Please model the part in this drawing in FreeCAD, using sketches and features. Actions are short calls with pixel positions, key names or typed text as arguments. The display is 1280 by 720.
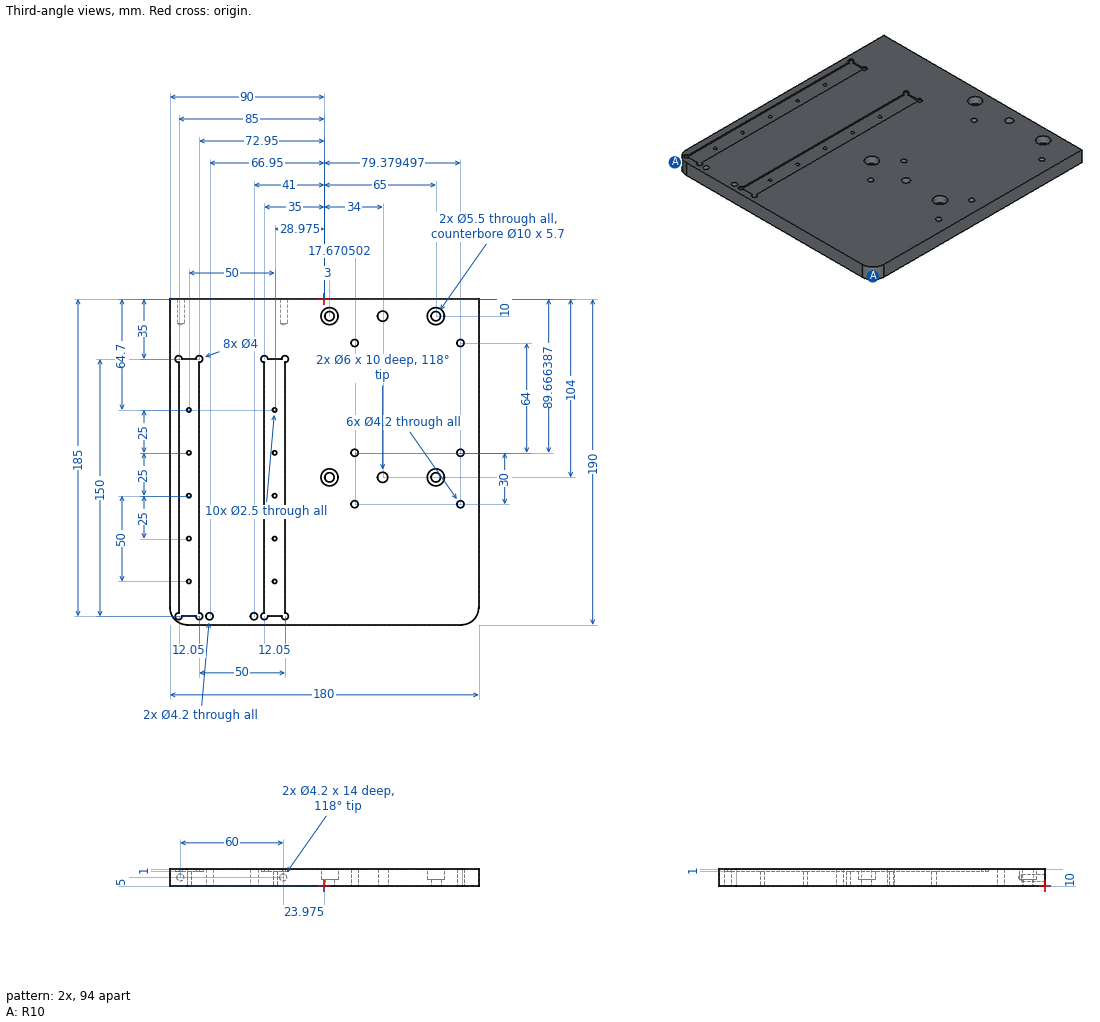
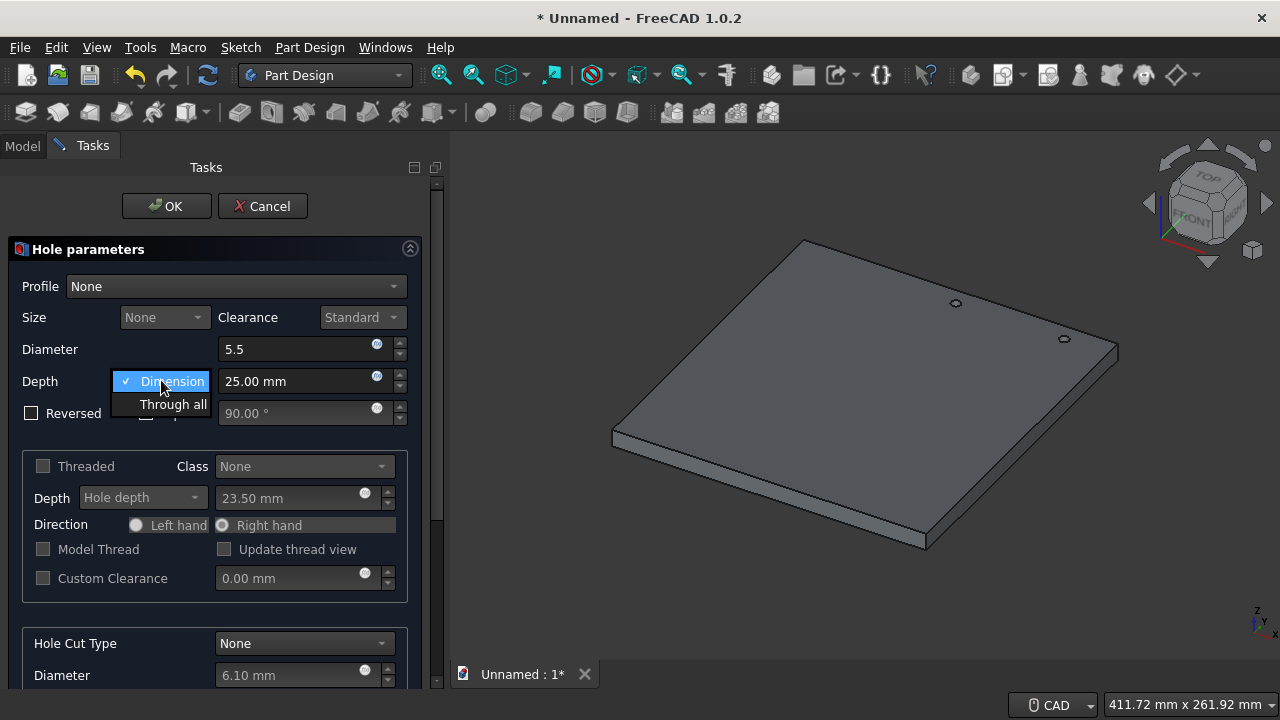
click(160, 404)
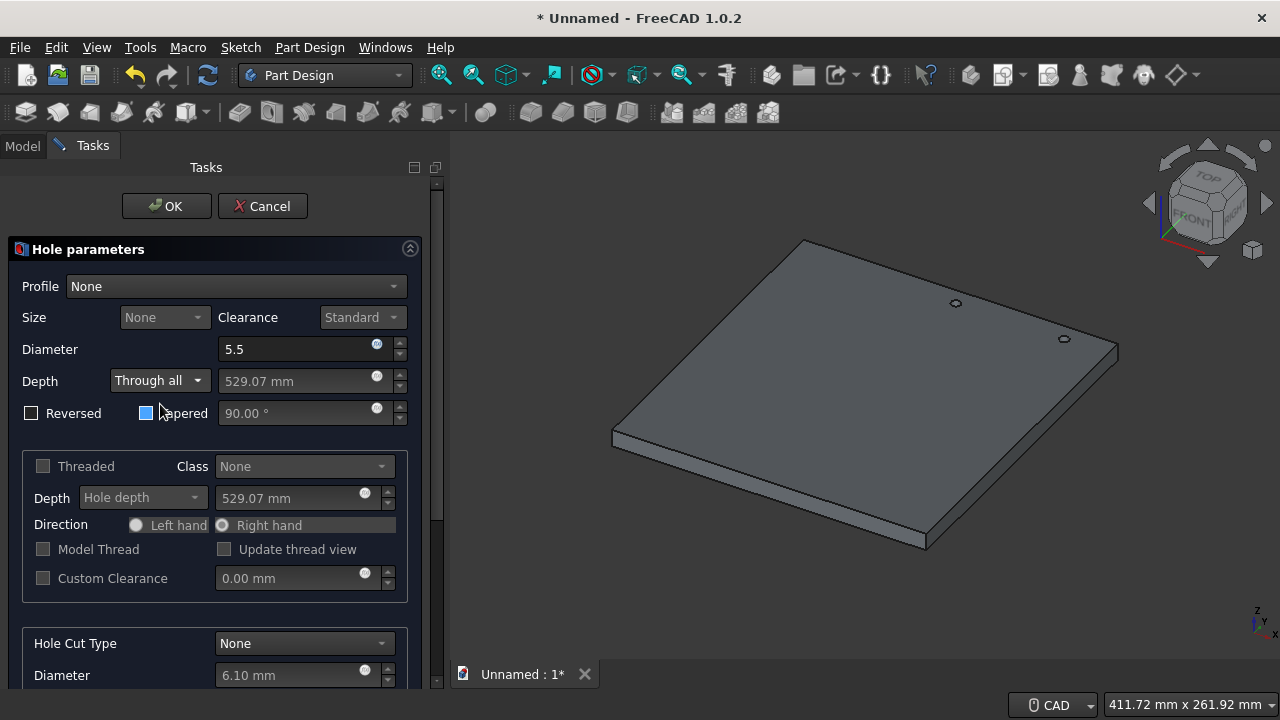
click(306, 644)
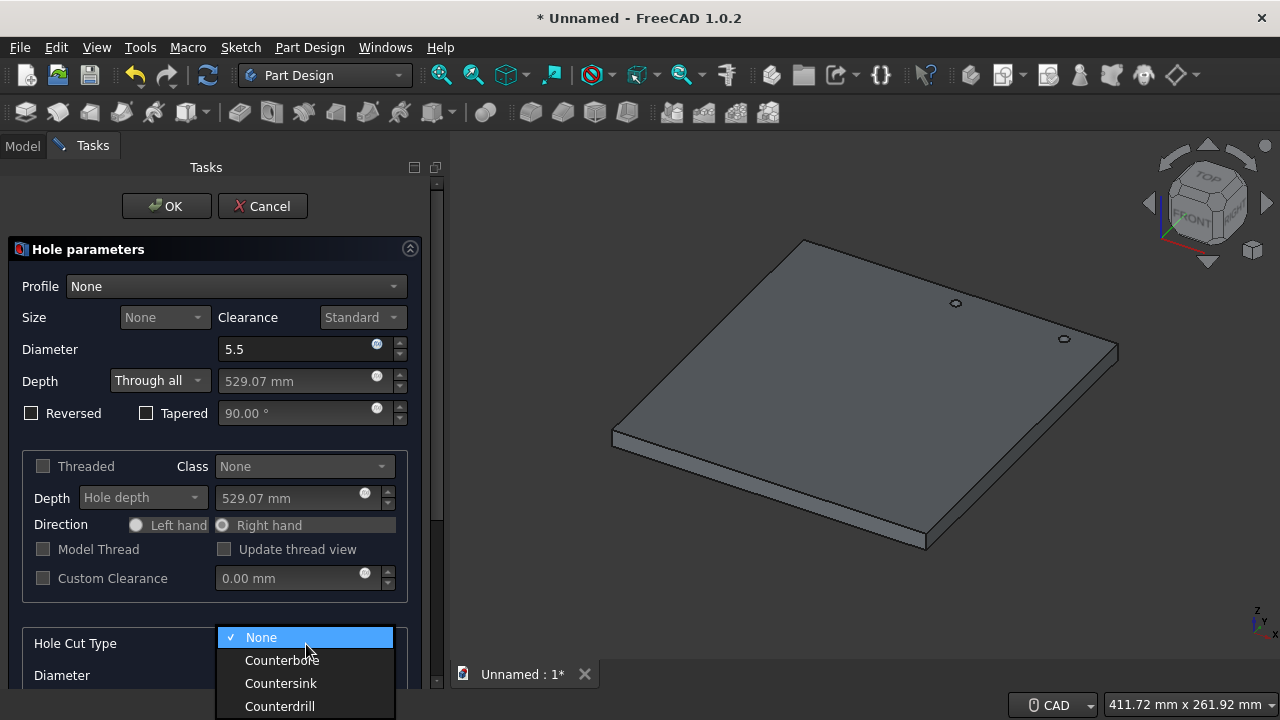
click(304, 660)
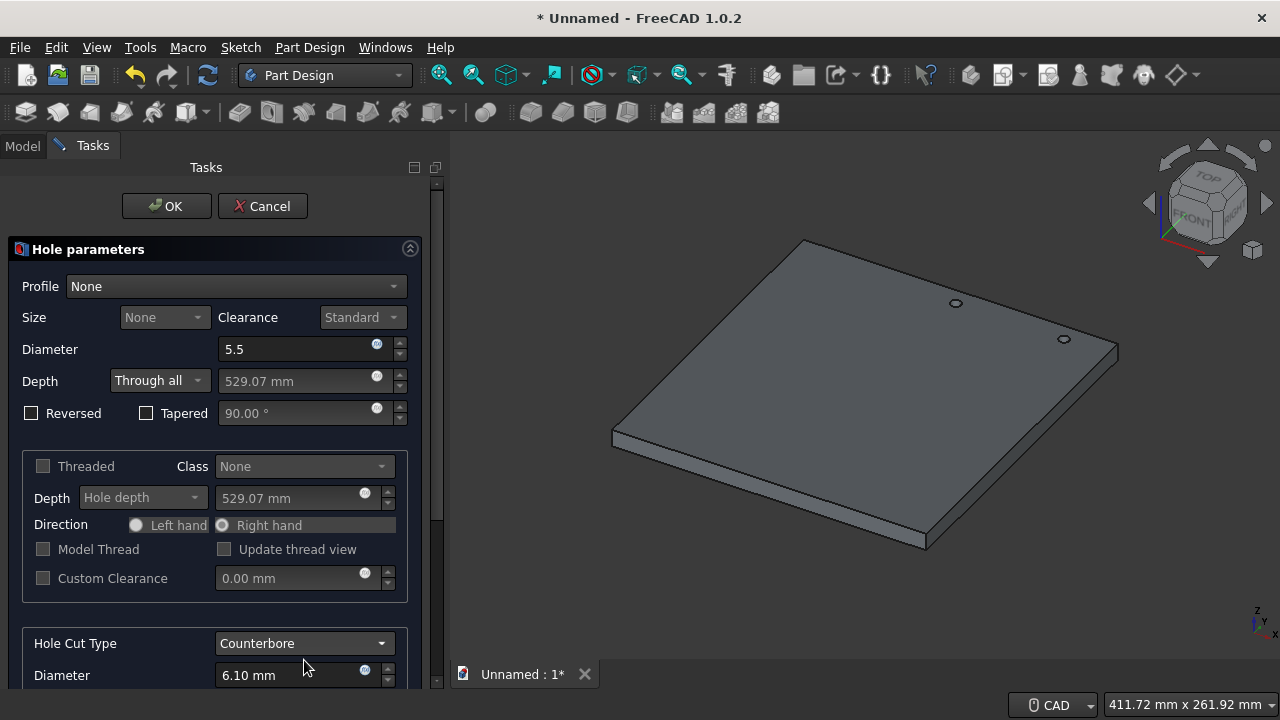
triple_click(298, 675)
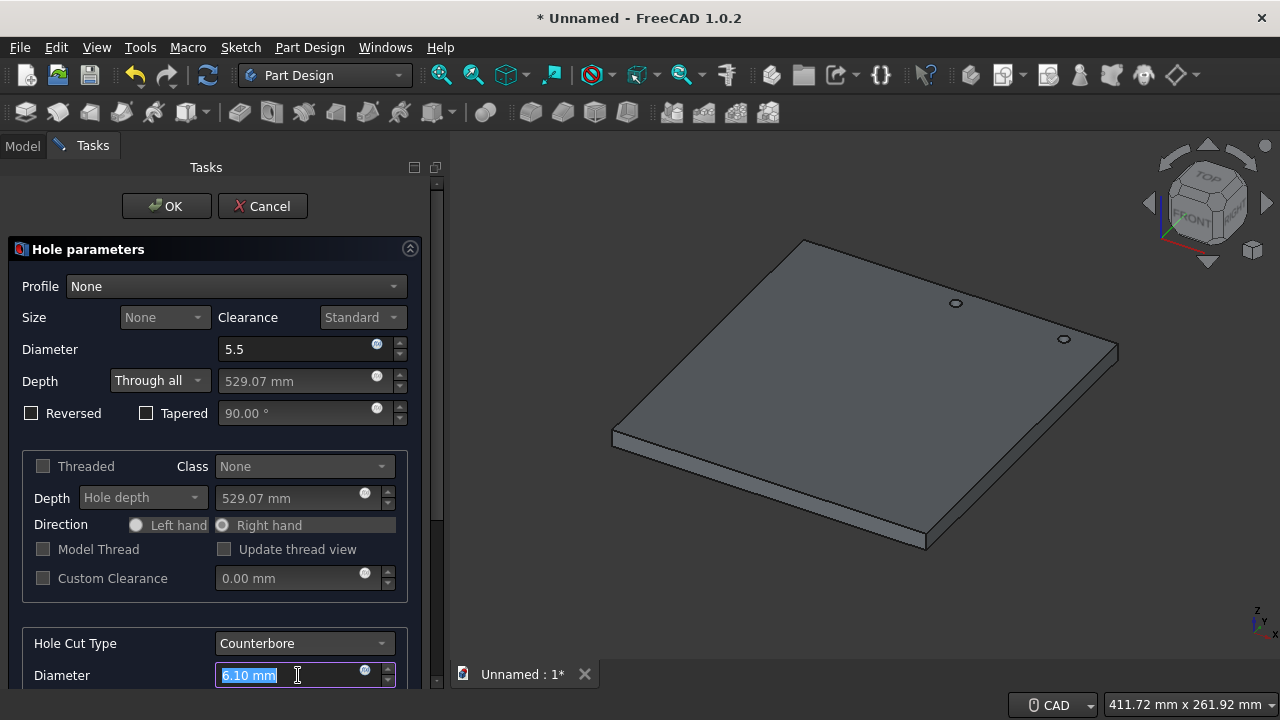
text(10)
key(Tab)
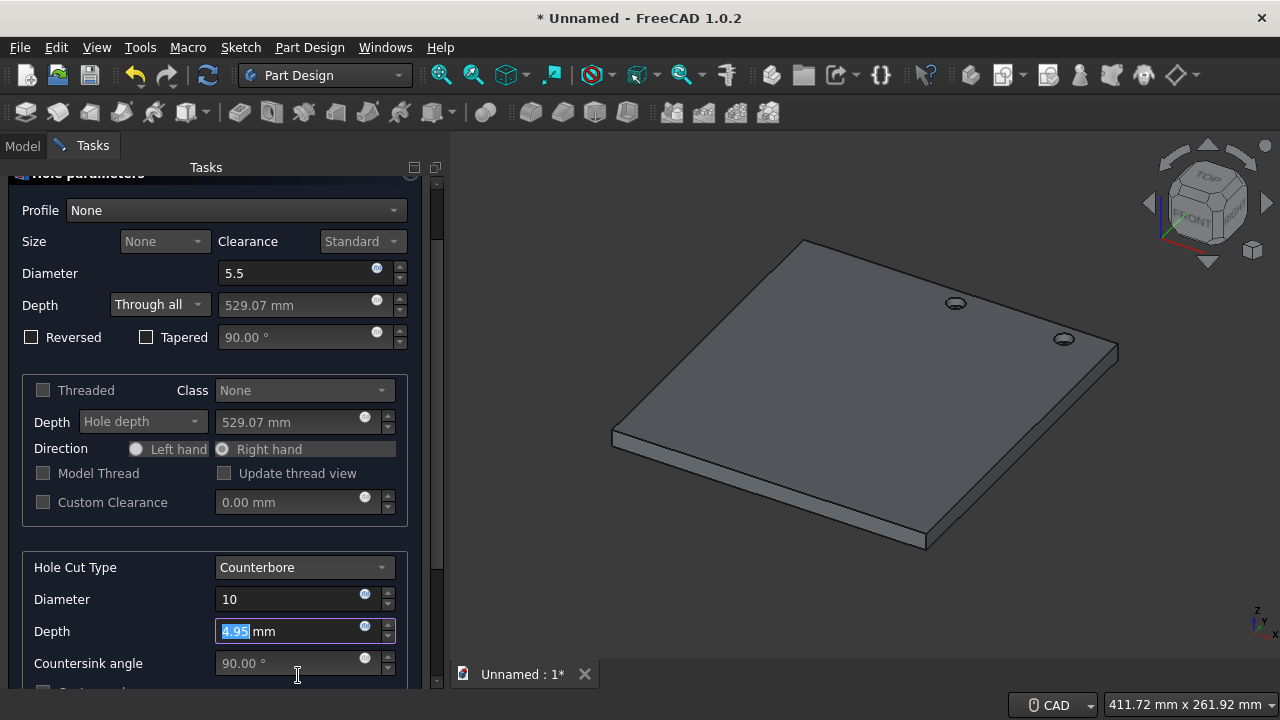
text(5.7)
key(Tab)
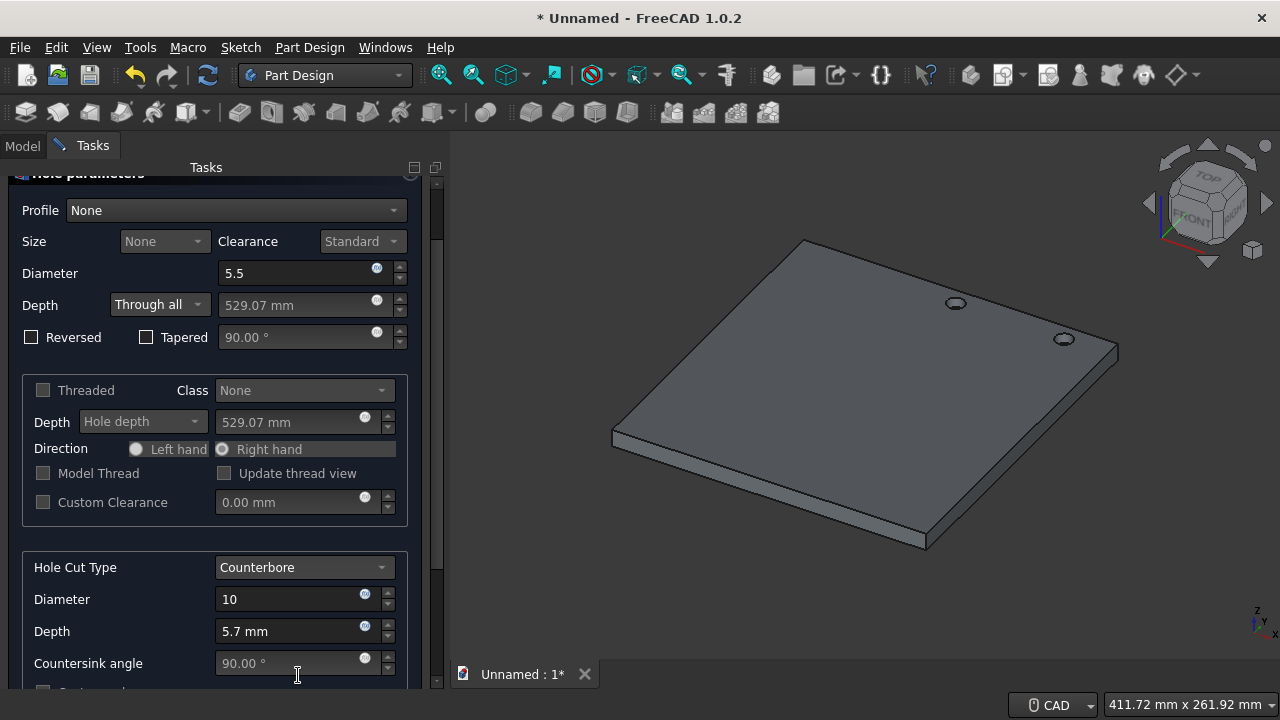
scroll(437, 432, up, 3)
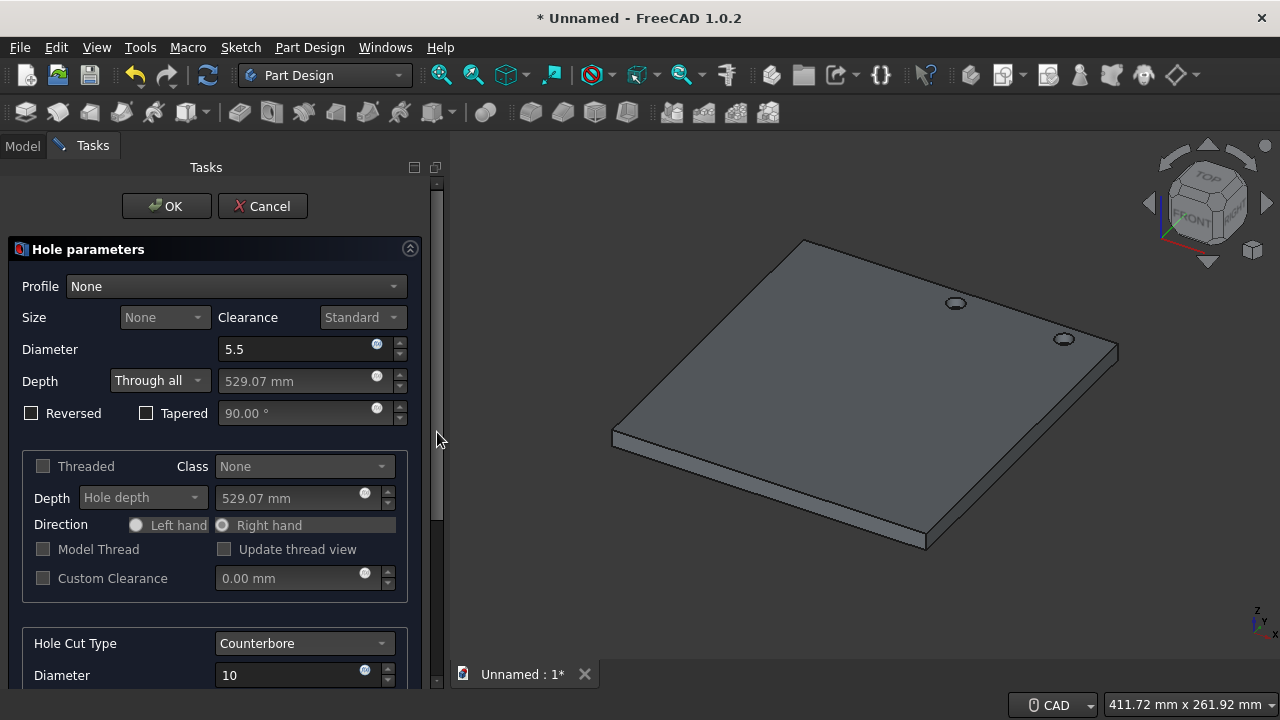
click(167, 206)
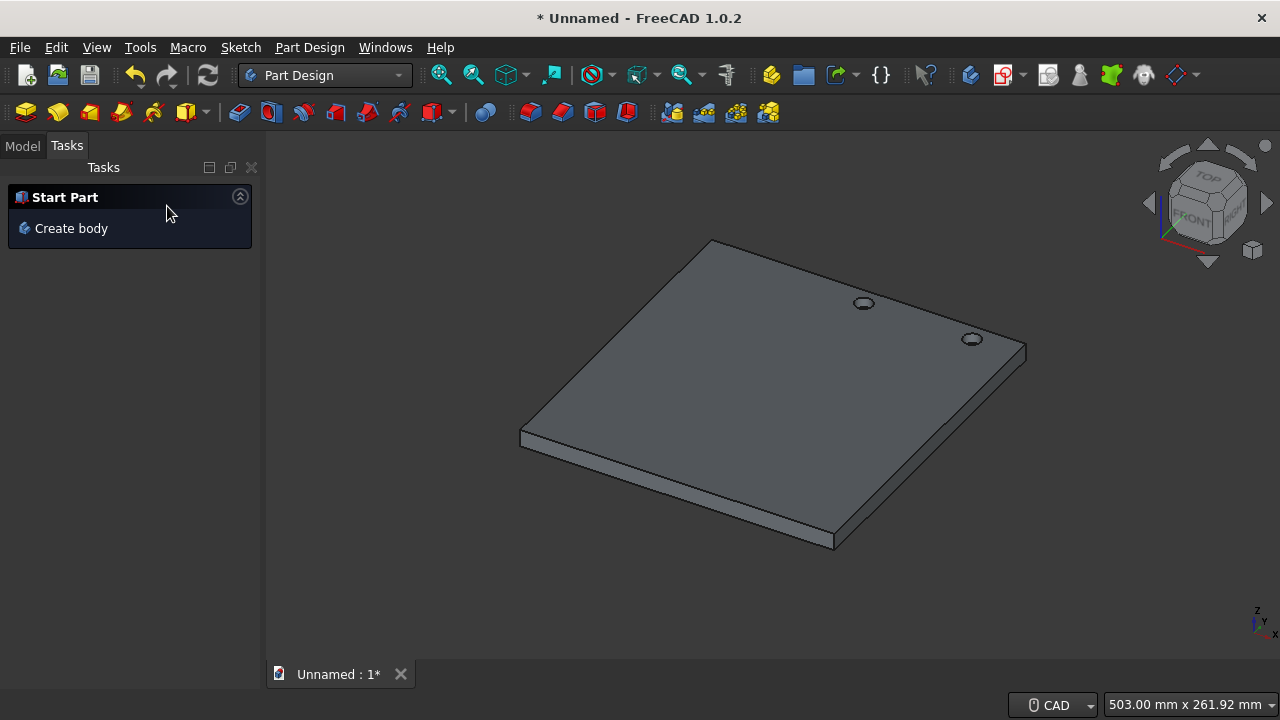
click(23, 145)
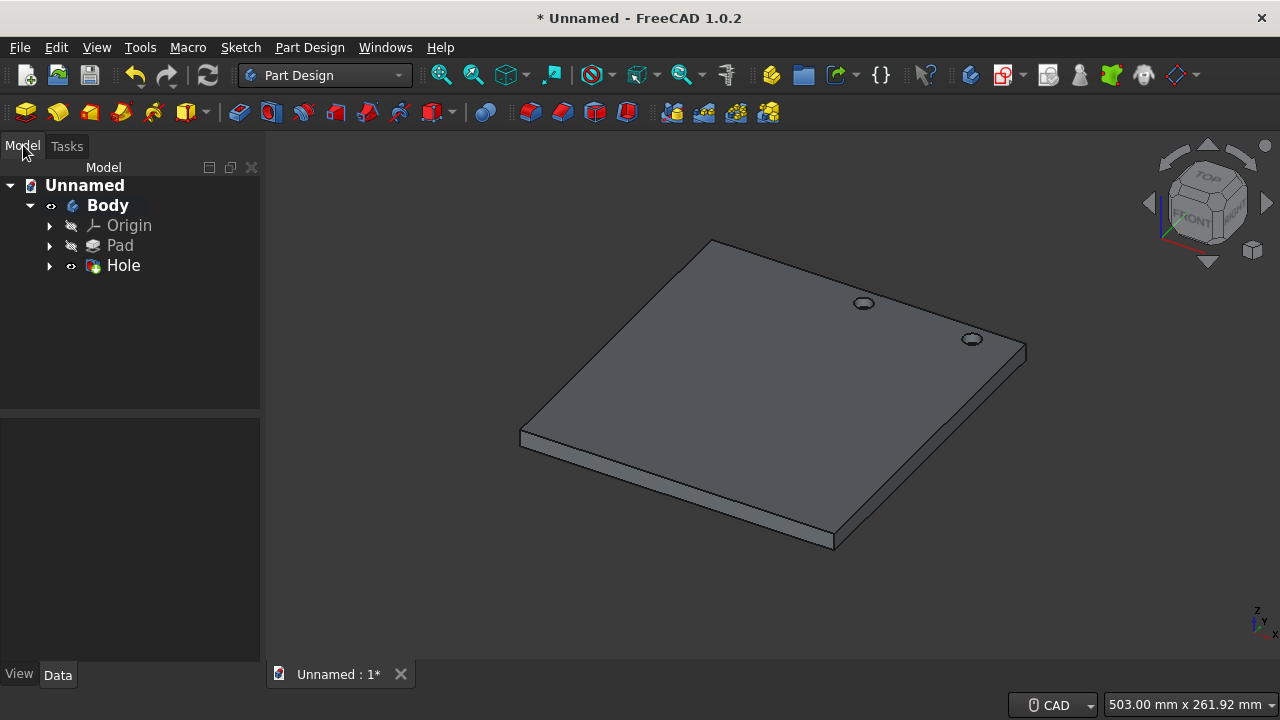
click(116, 266)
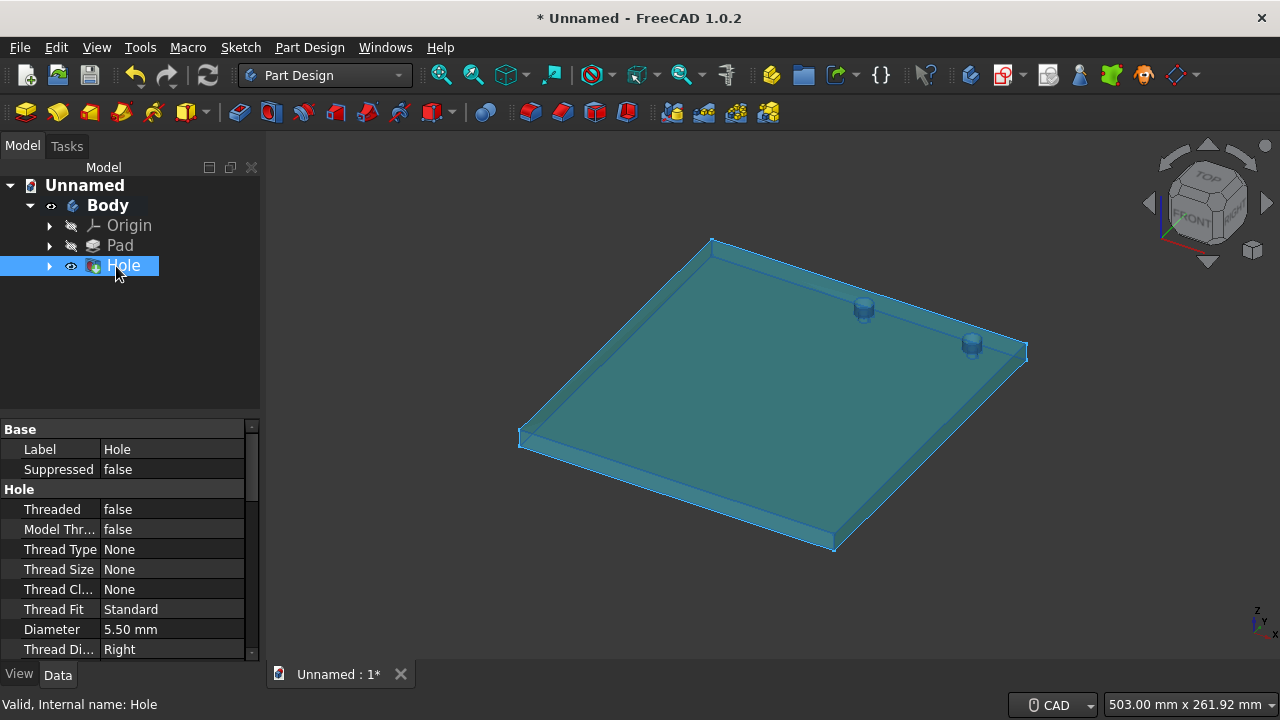
click(704, 112)